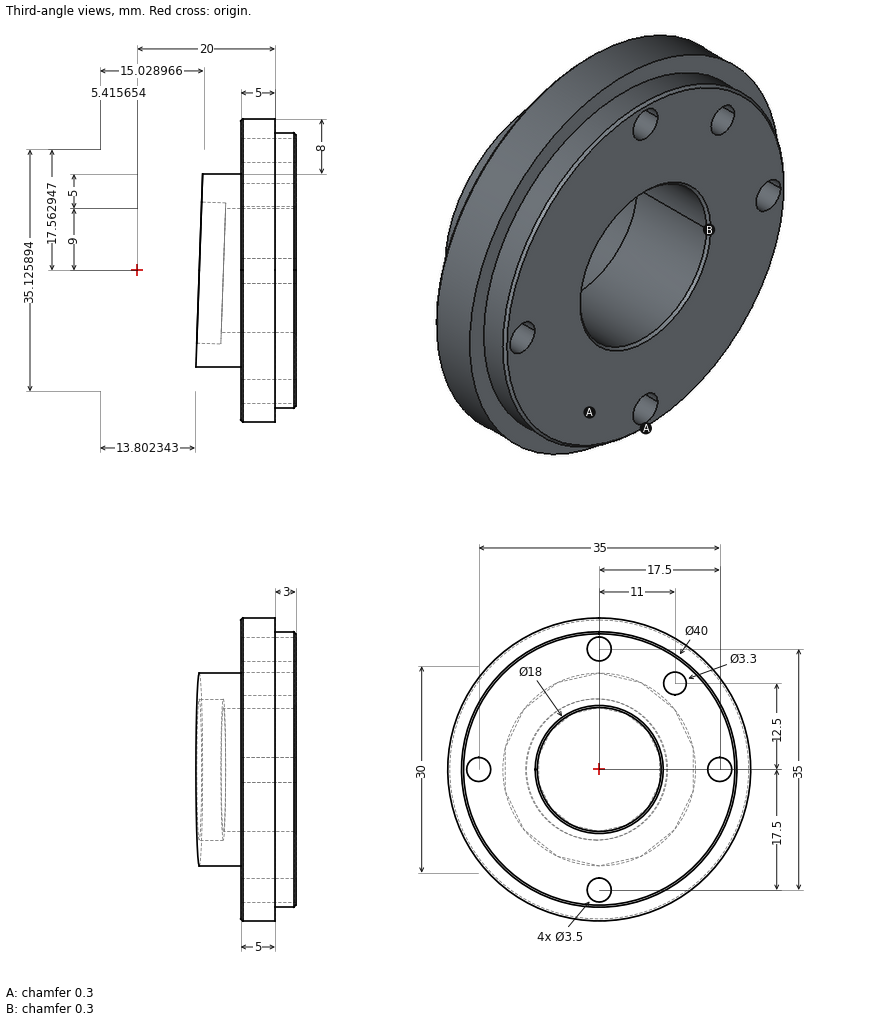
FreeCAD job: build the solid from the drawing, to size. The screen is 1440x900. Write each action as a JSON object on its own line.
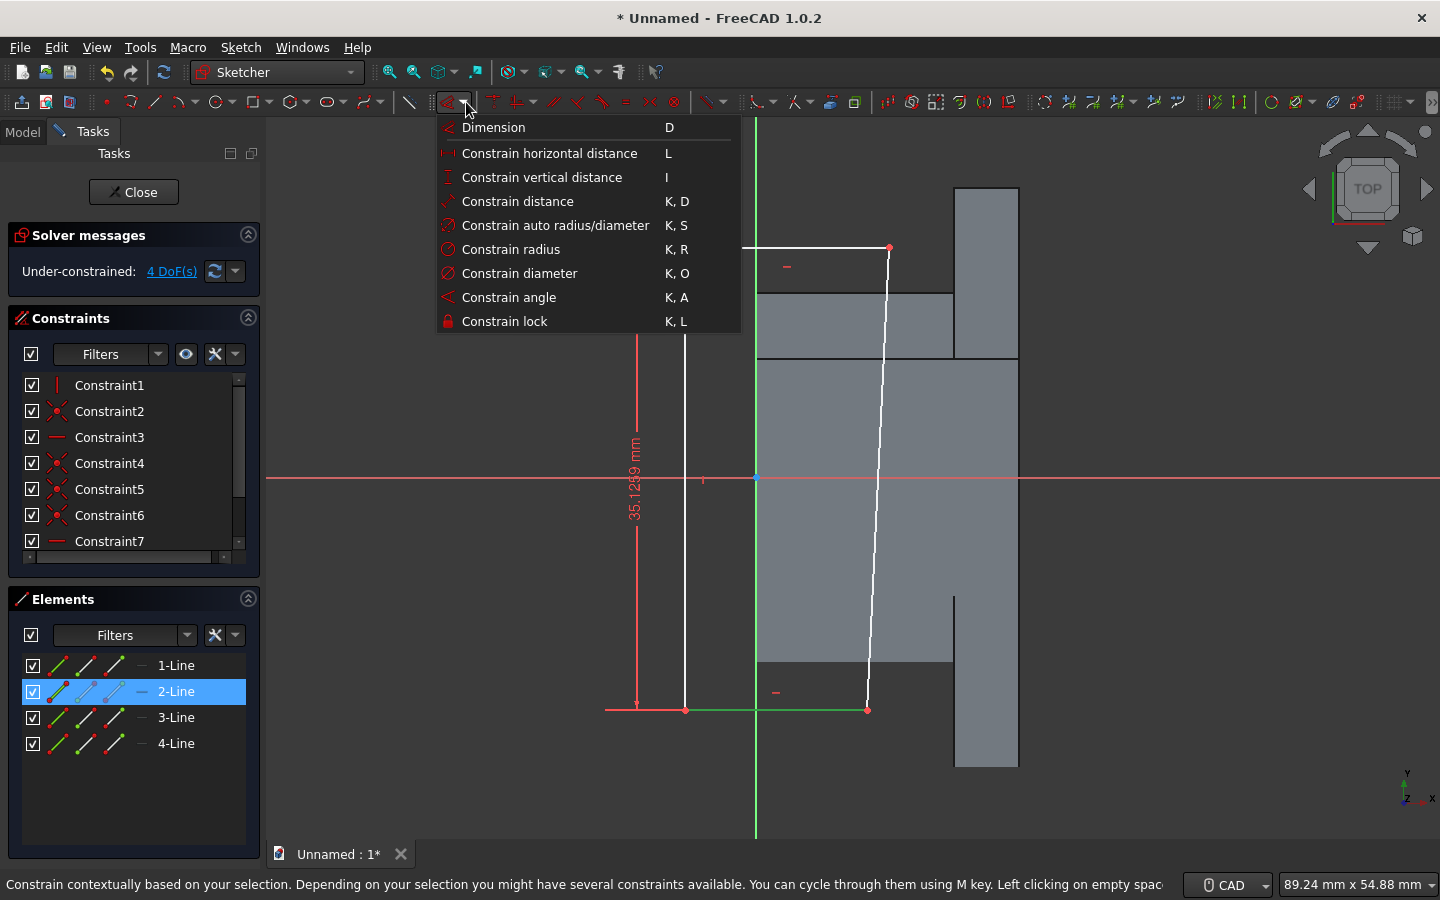
{"action": "left_click", "coordinate": [589, 153]}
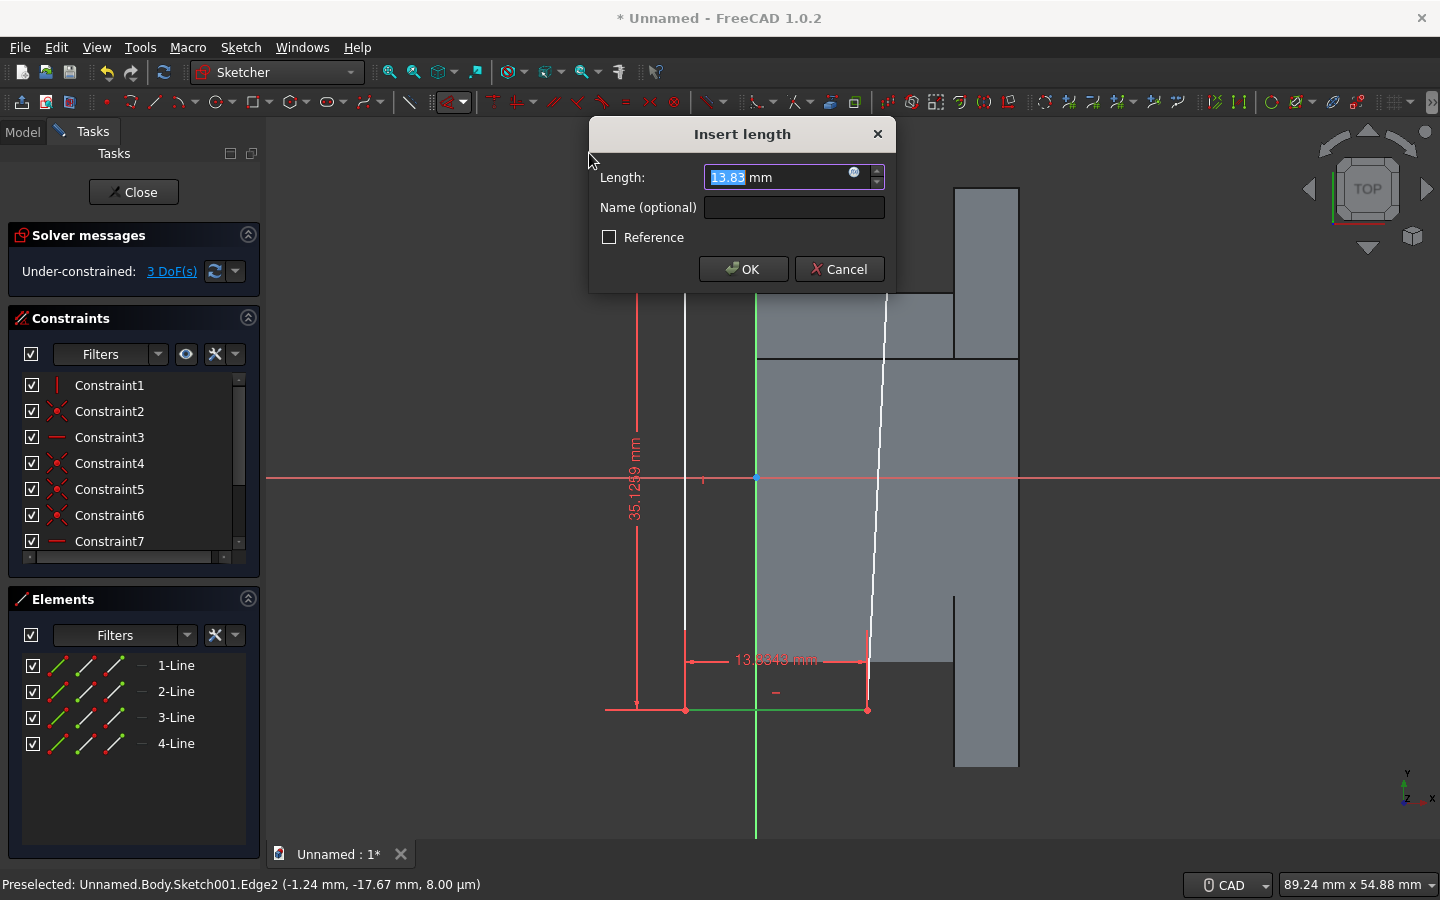
{"action": "type", "text": "13.802343"}
{"action": "key", "text": "Return"}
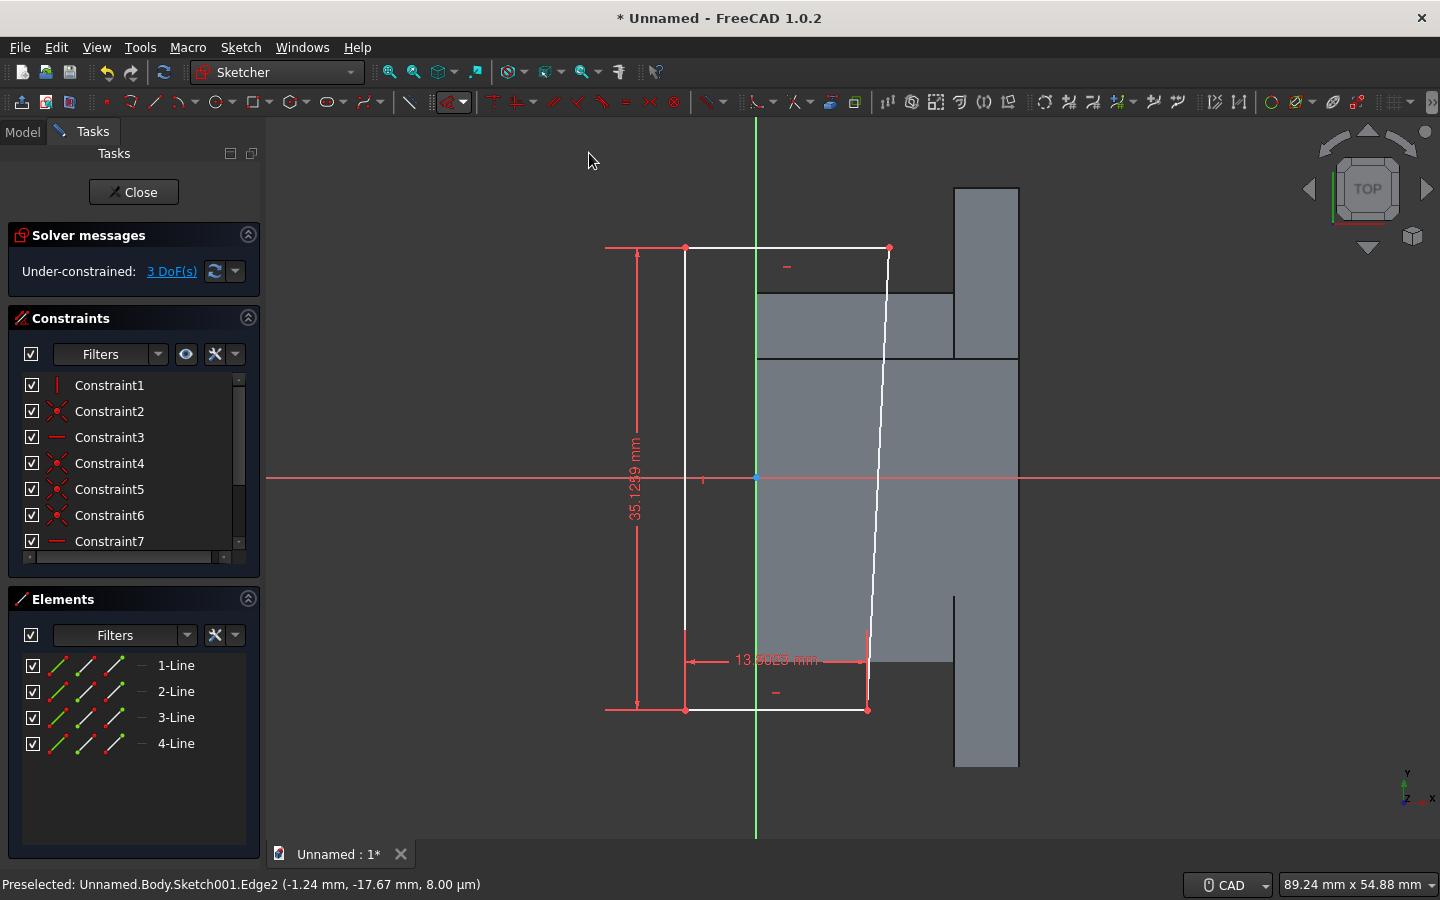
{"action": "left_click", "coordinate": [828, 248]}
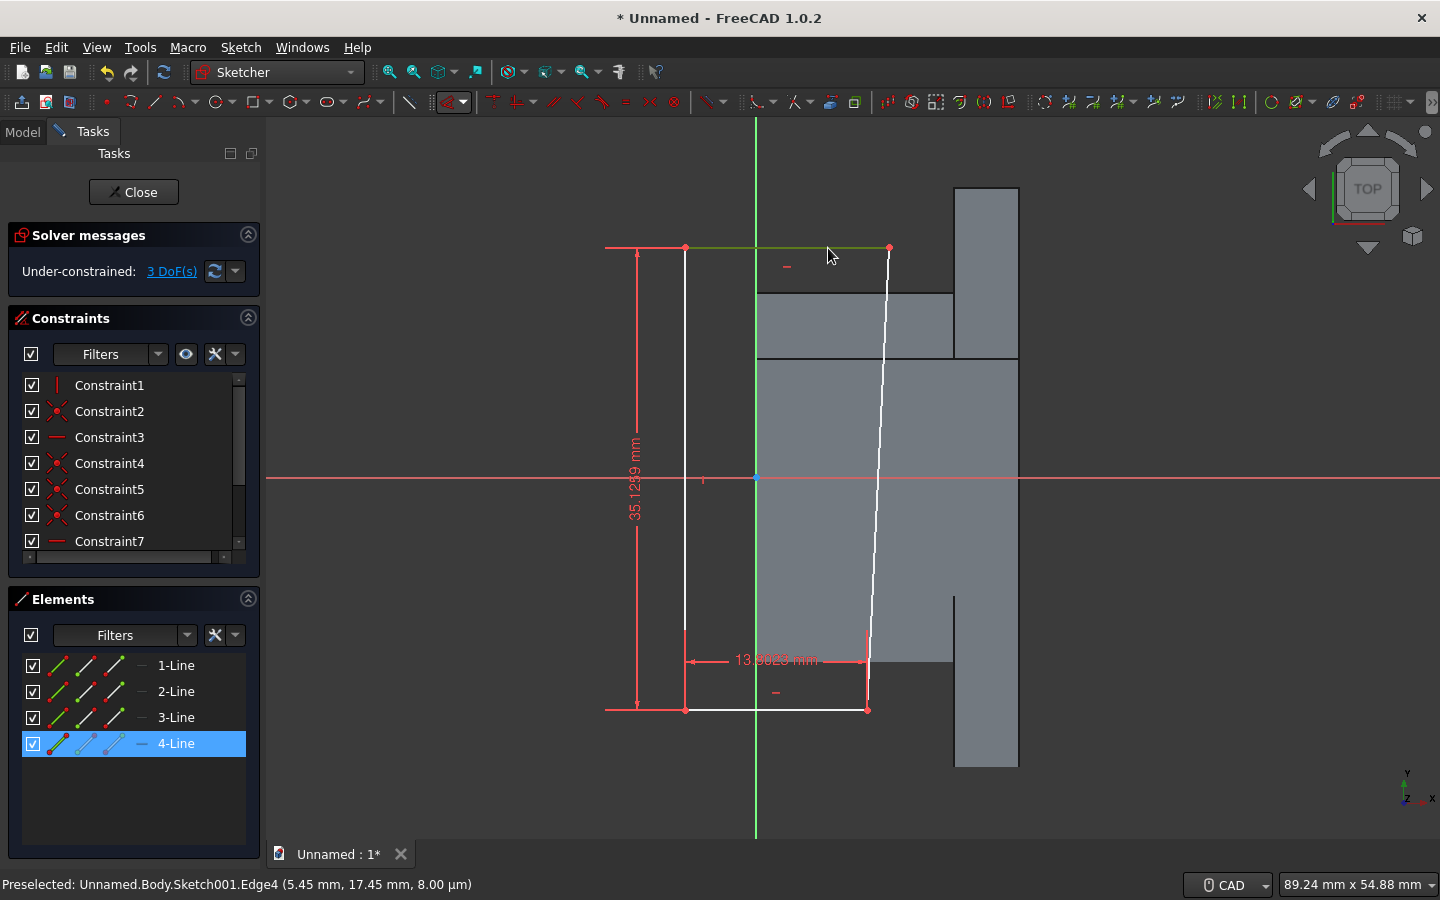
{"action": "left_click", "coordinate": [466, 102]}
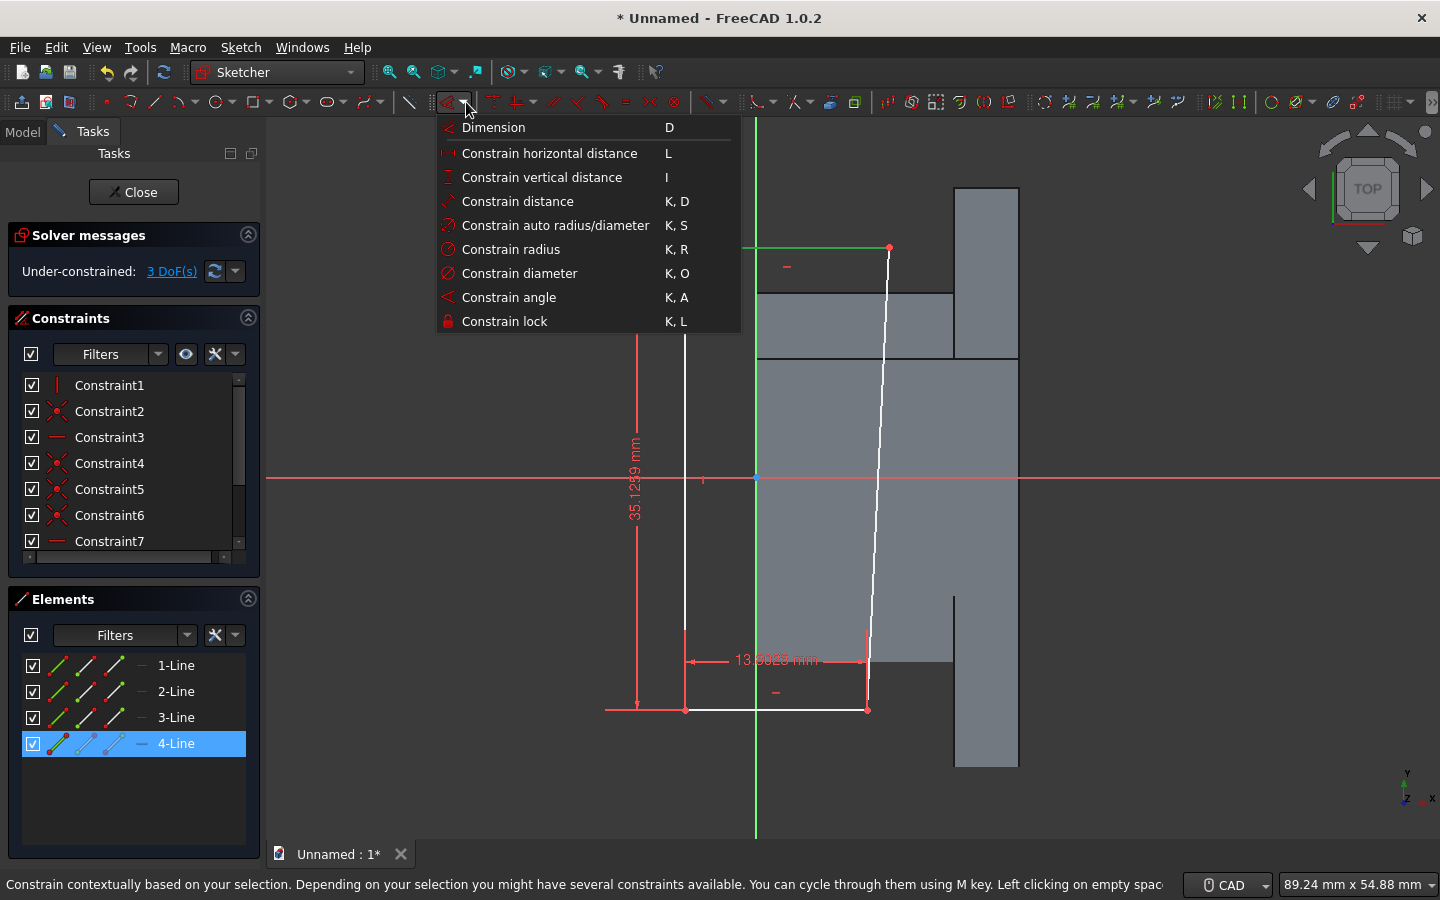
{"action": "left_click", "coordinate": [589, 153]}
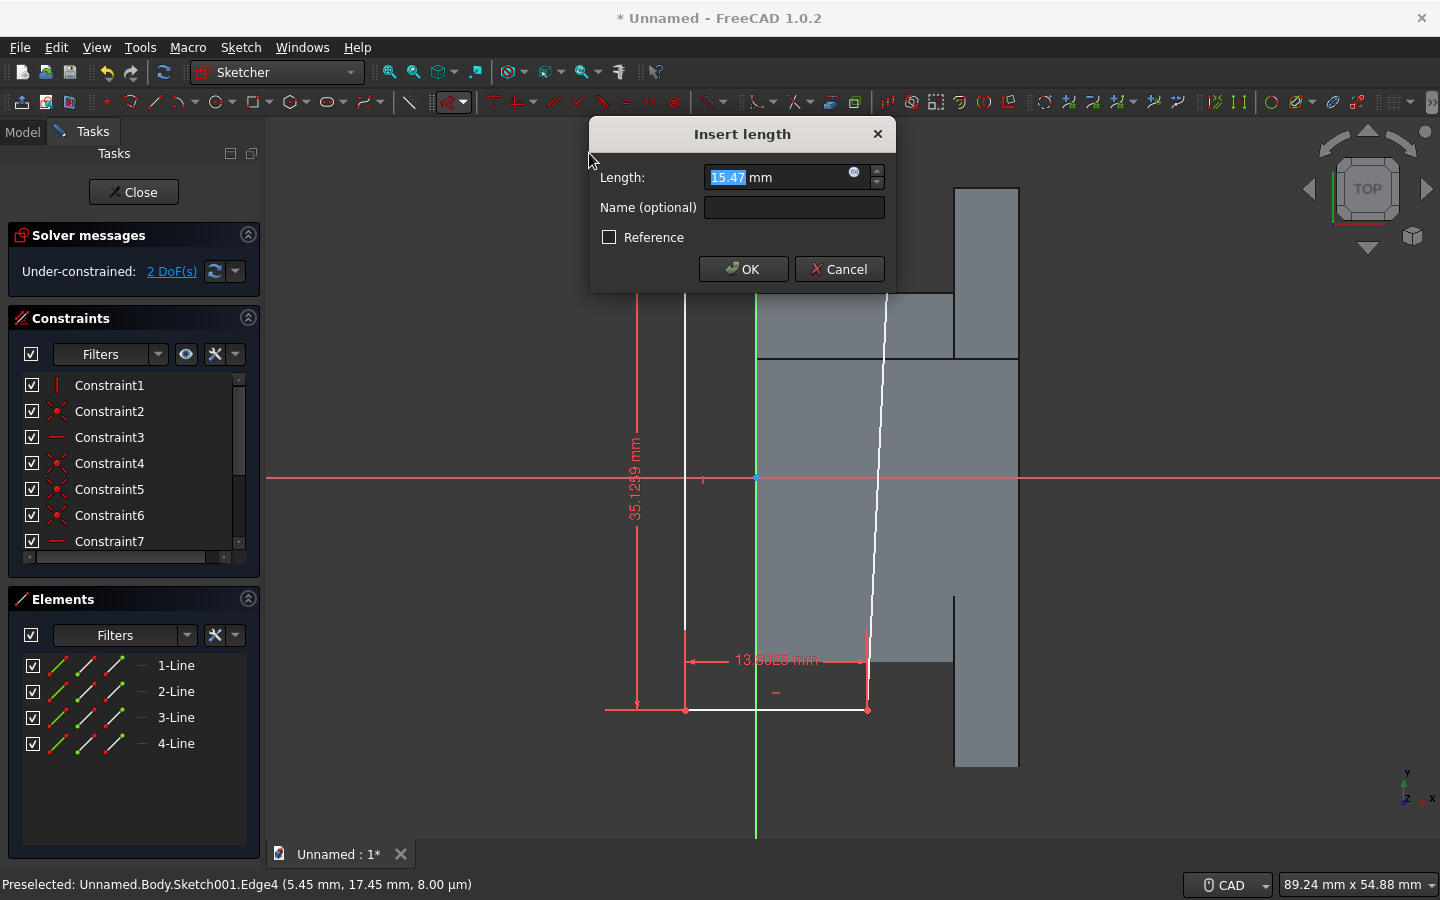
{"action": "type", "text": "15.028966"}
{"action": "key", "text": "Return"}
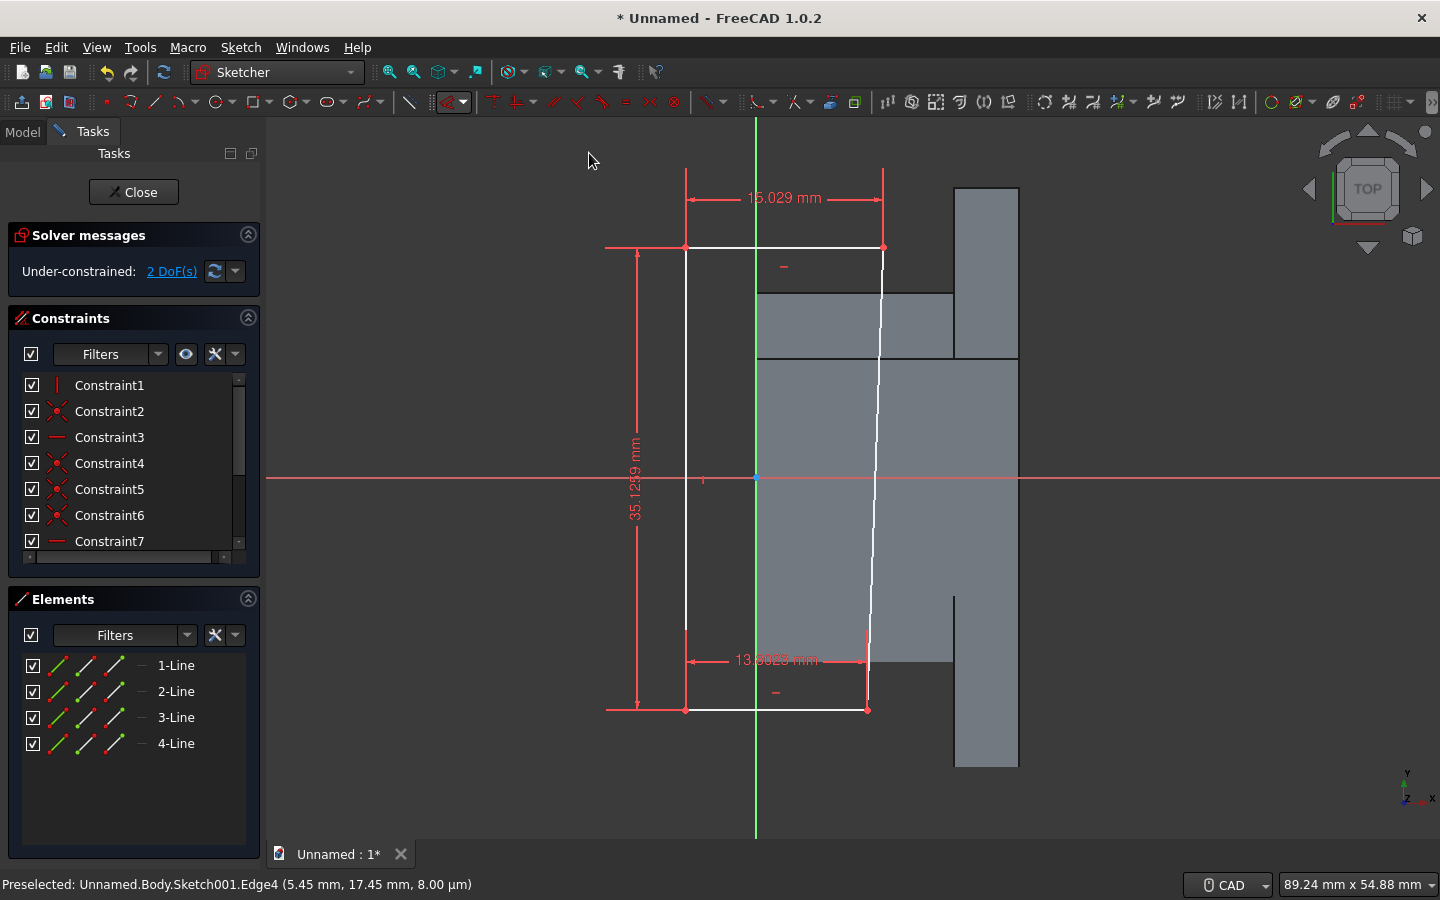
{"action": "left_click", "coordinate": [686, 248]}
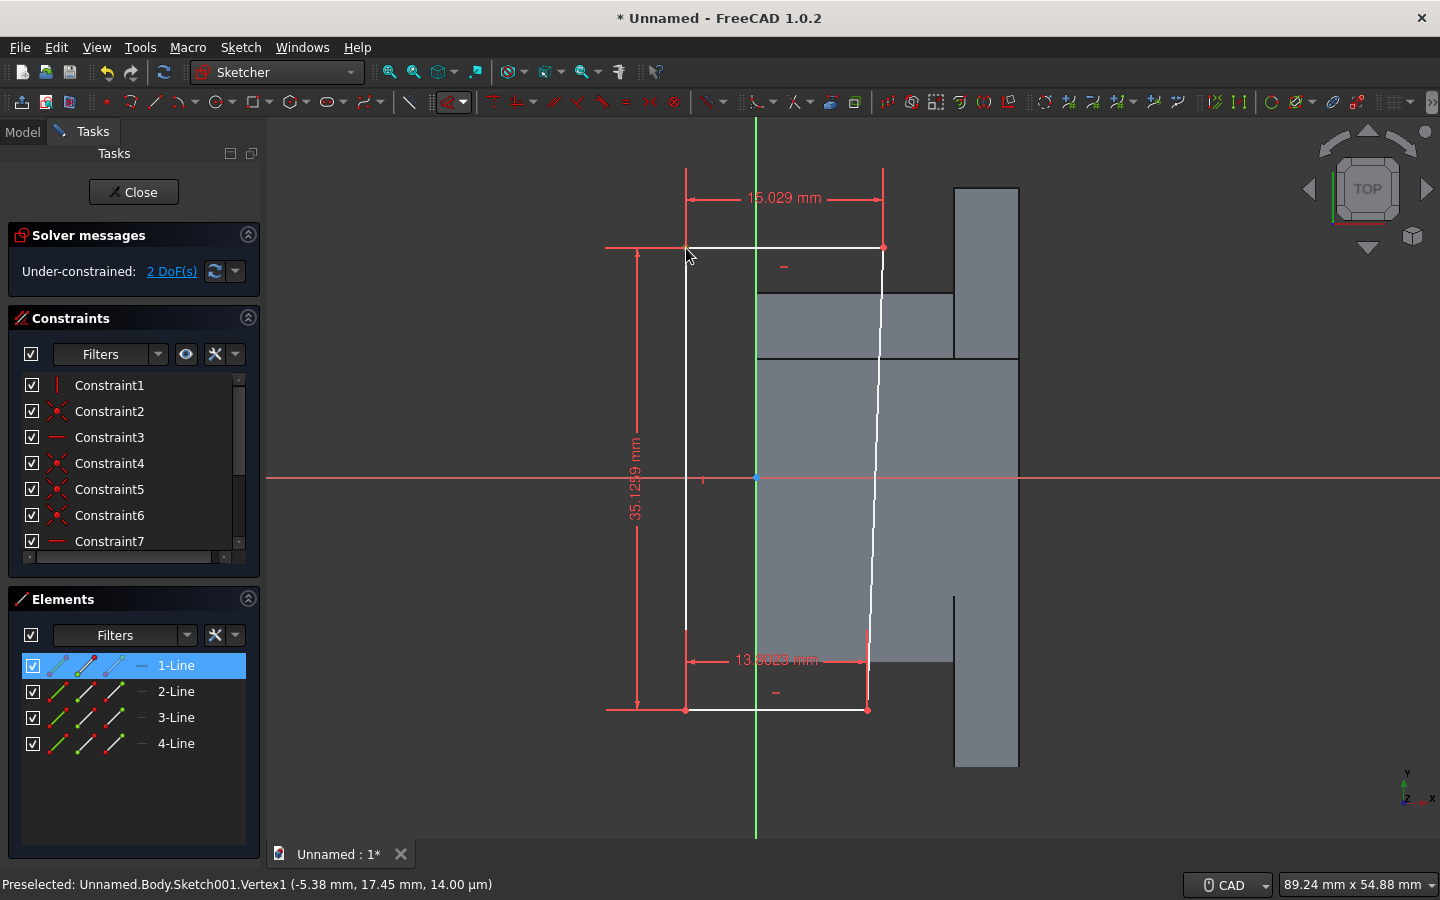
{"action": "key", "text": "l"}